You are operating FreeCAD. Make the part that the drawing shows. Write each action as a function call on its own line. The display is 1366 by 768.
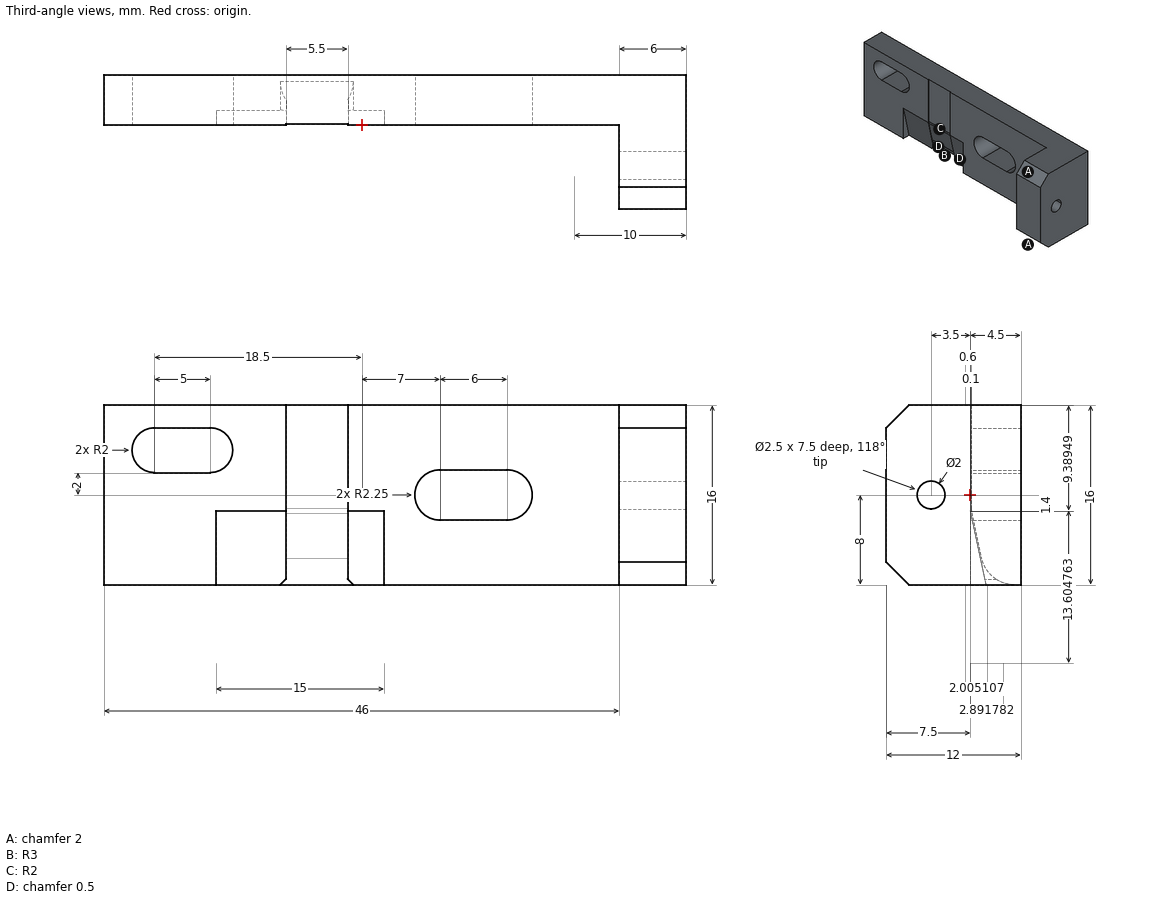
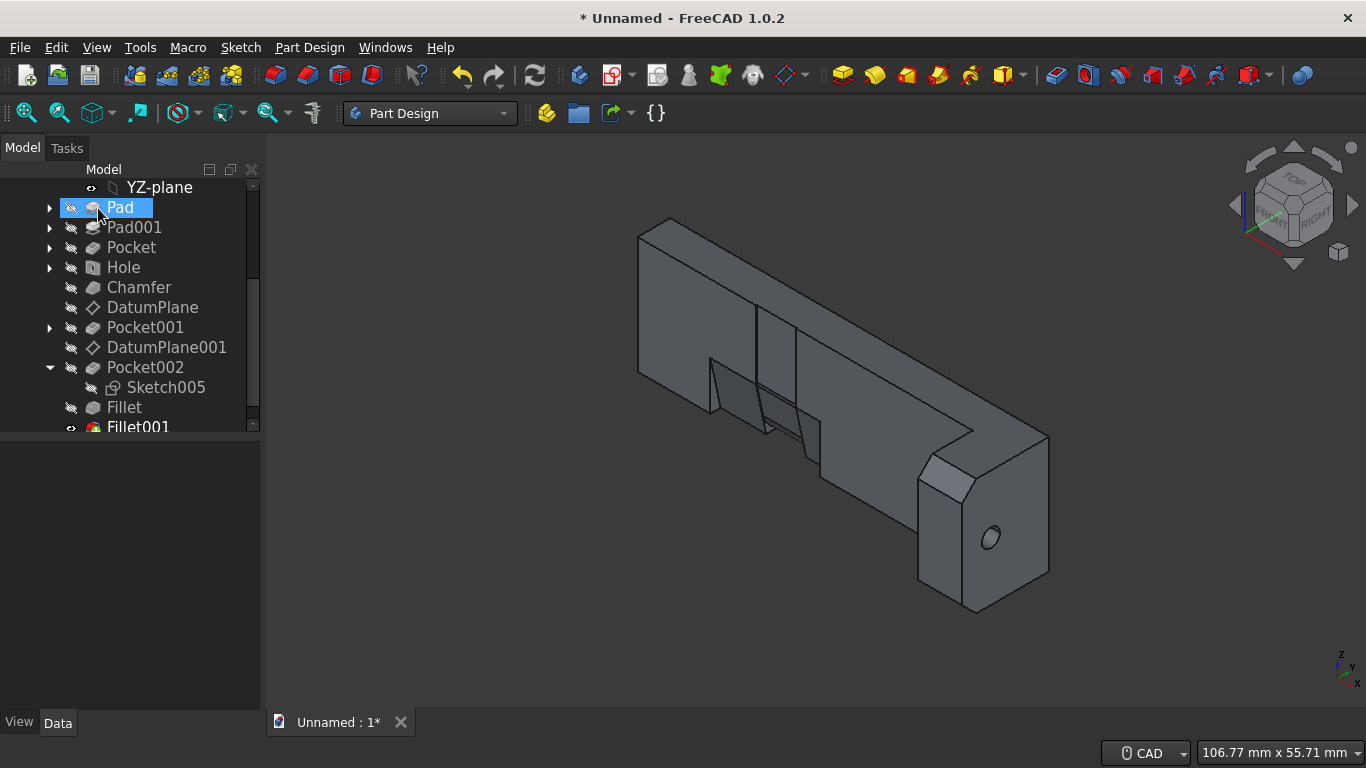
key(4)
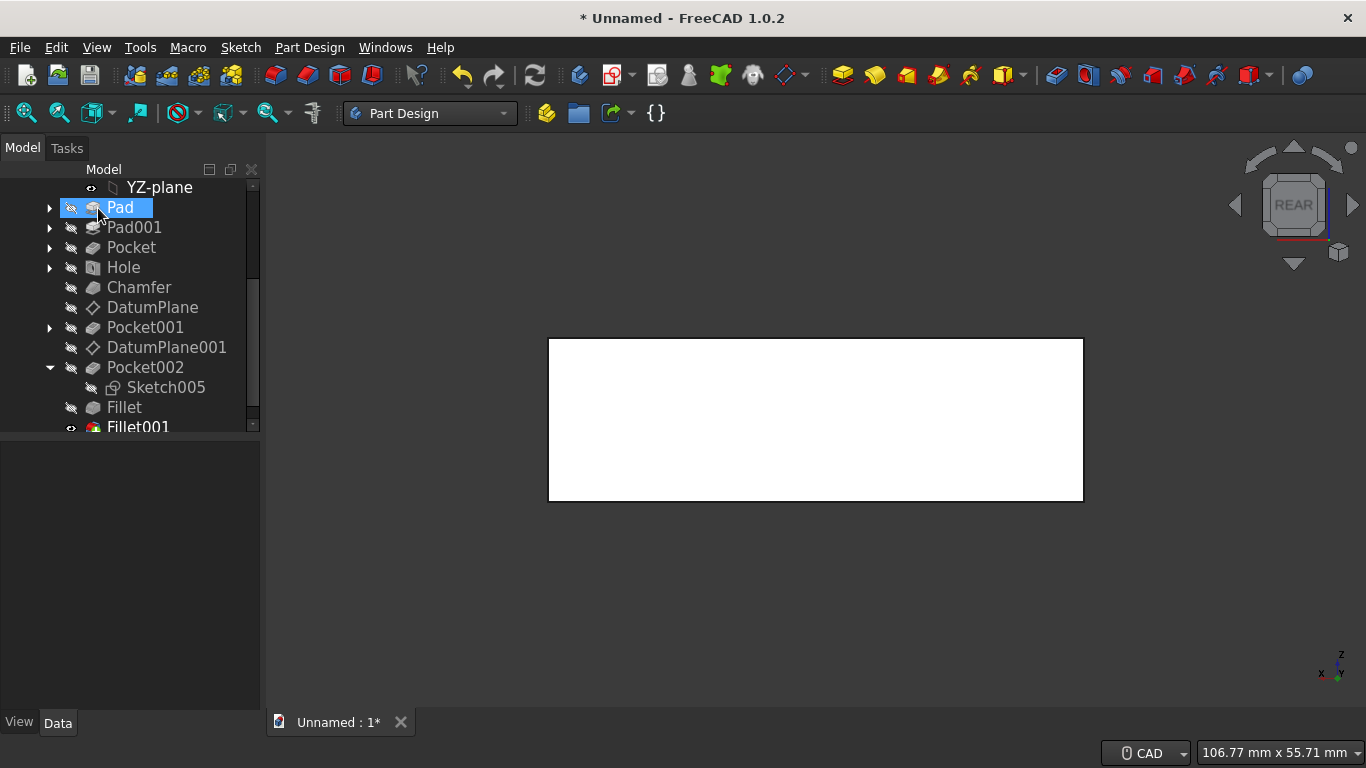
click(663, 419)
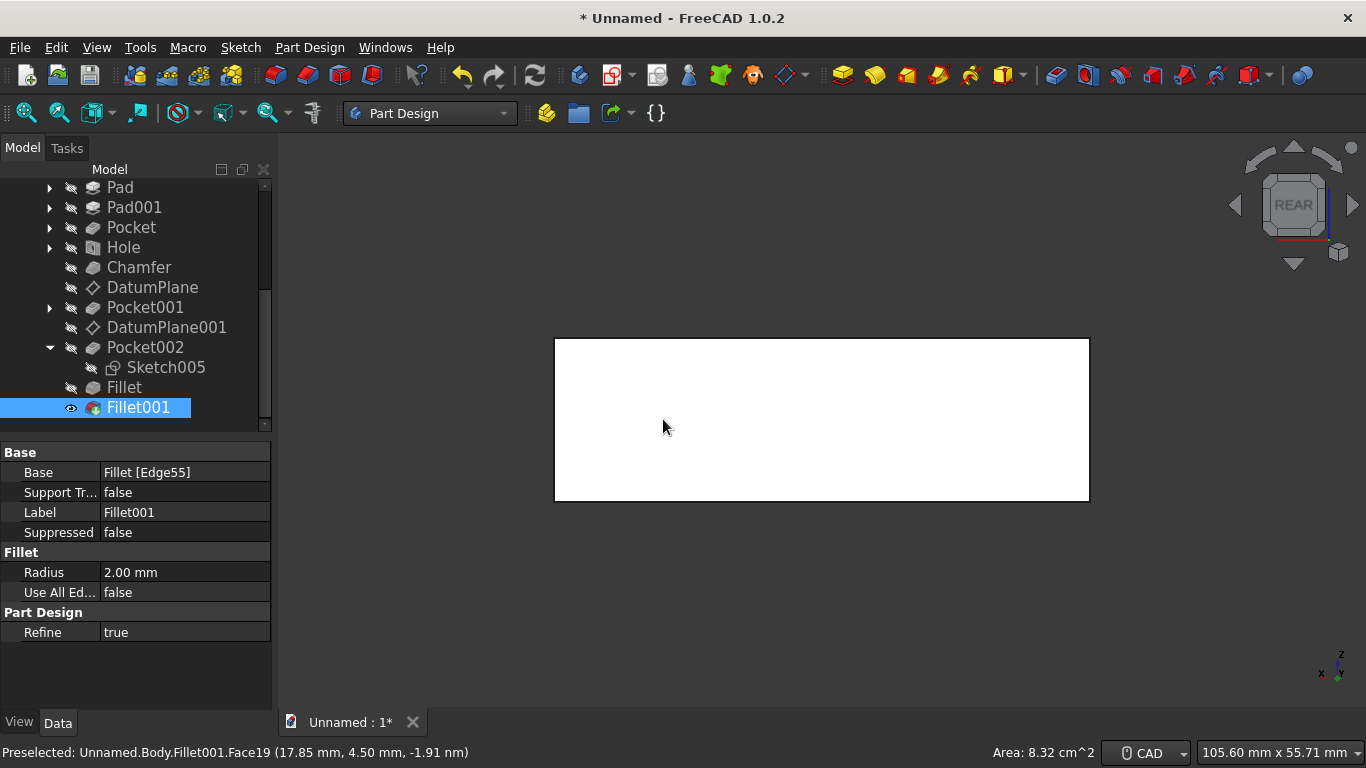
click(612, 76)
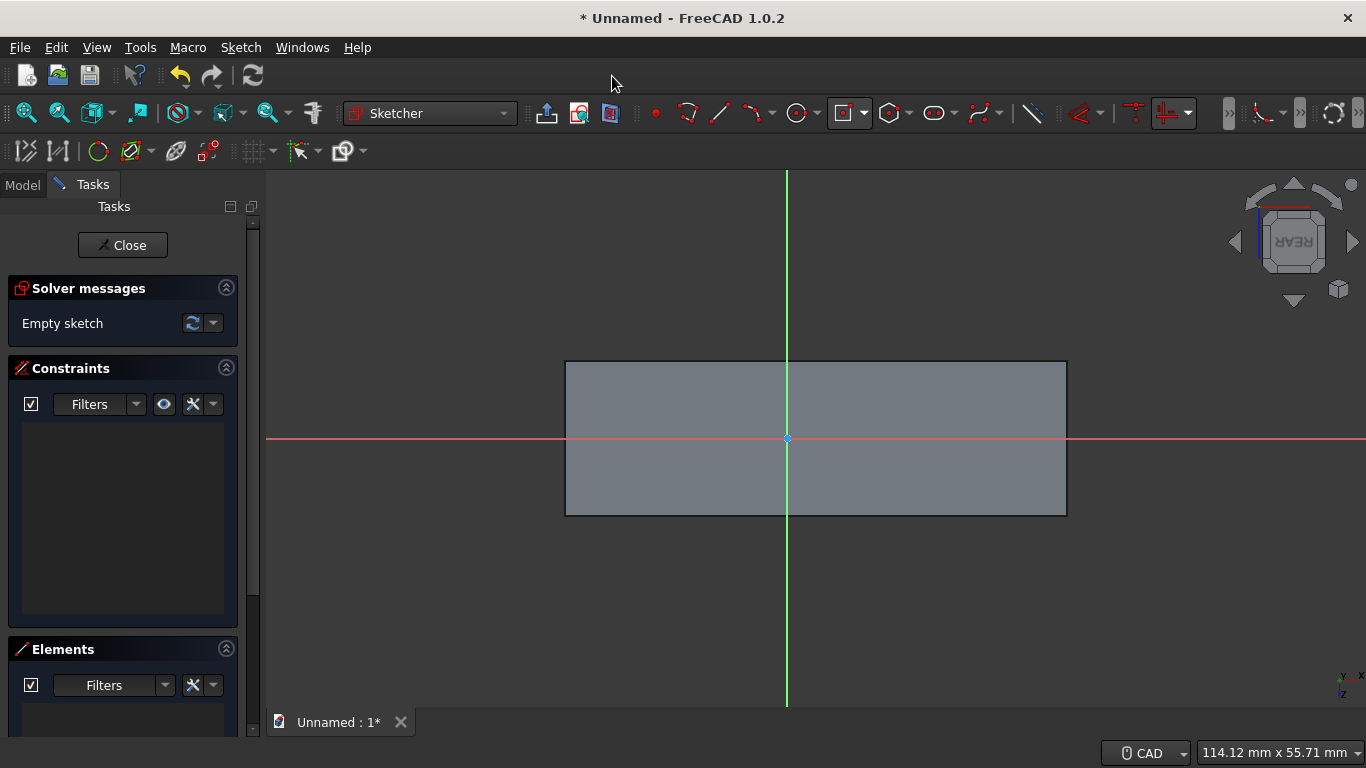
scroll(663, 480, up, 6)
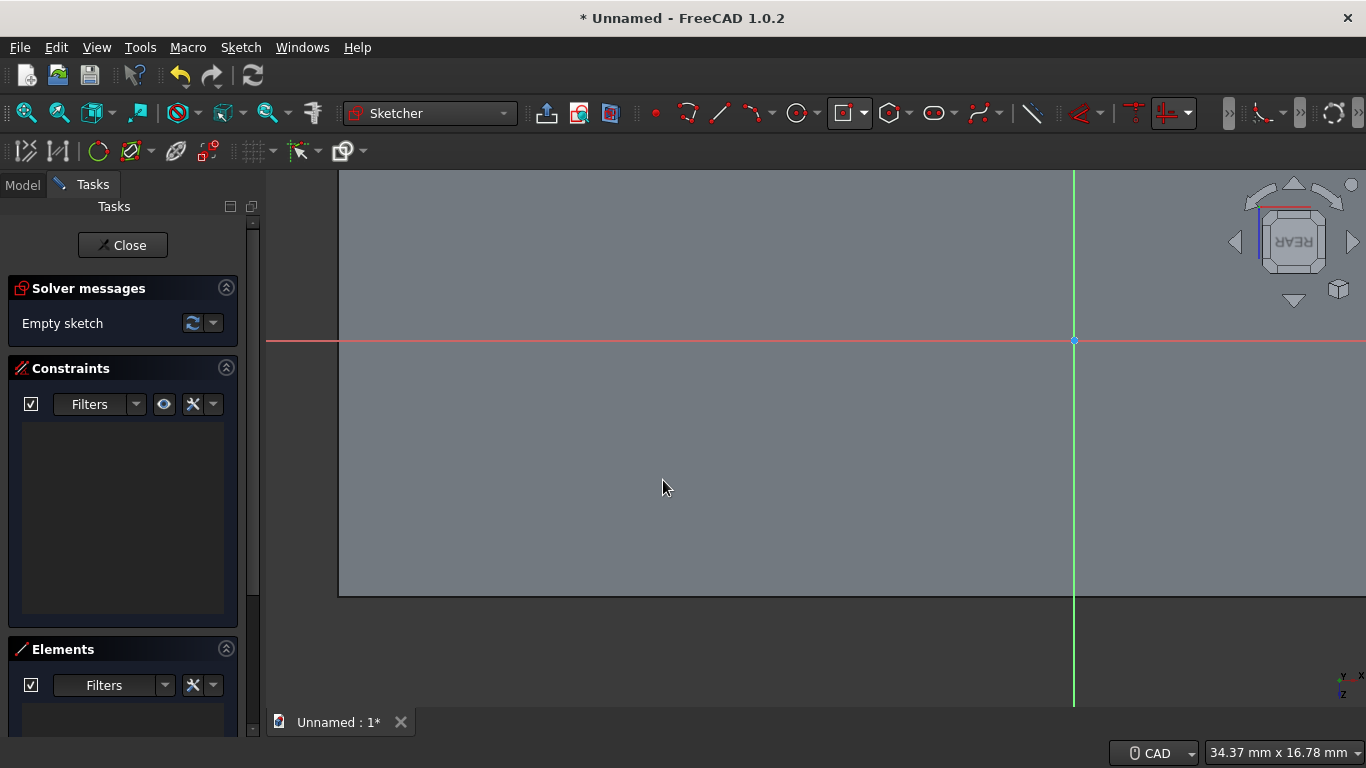
key(g)
key(s)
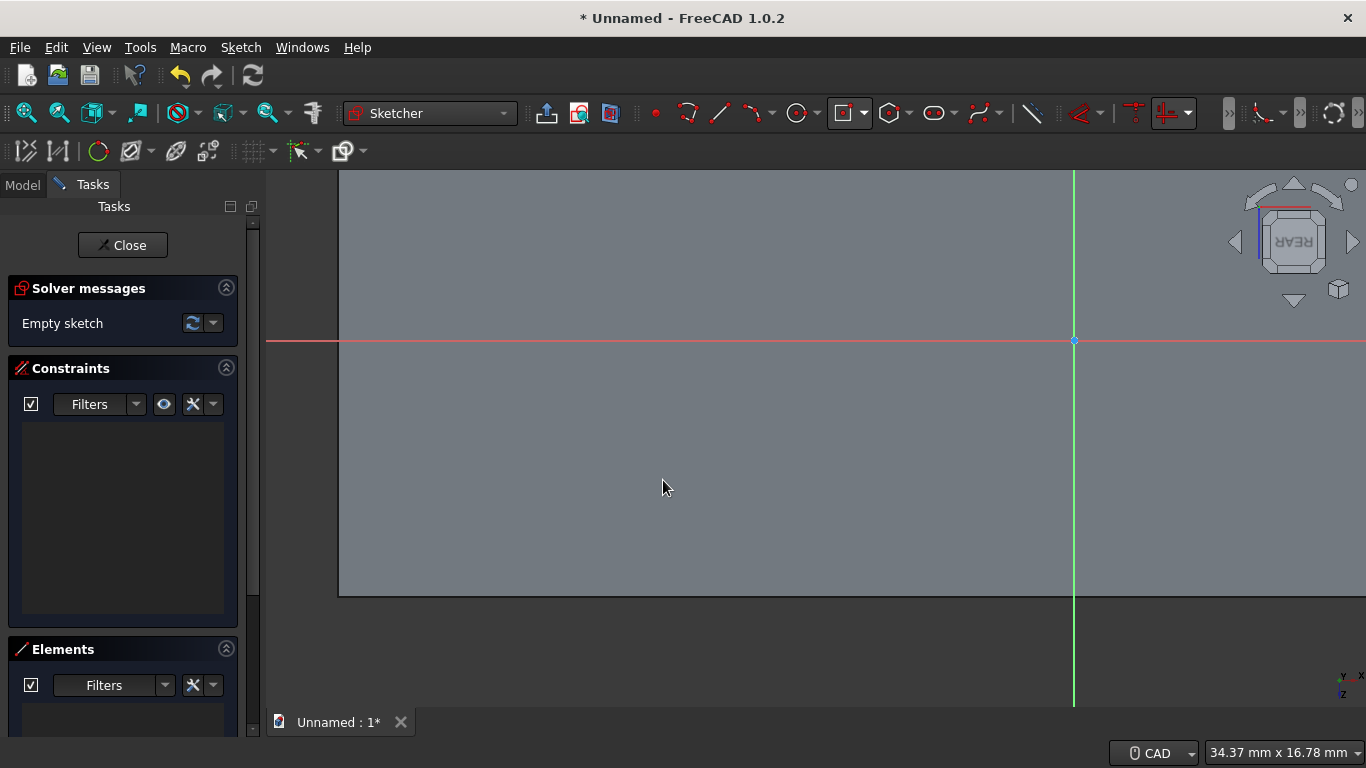
click(482, 469)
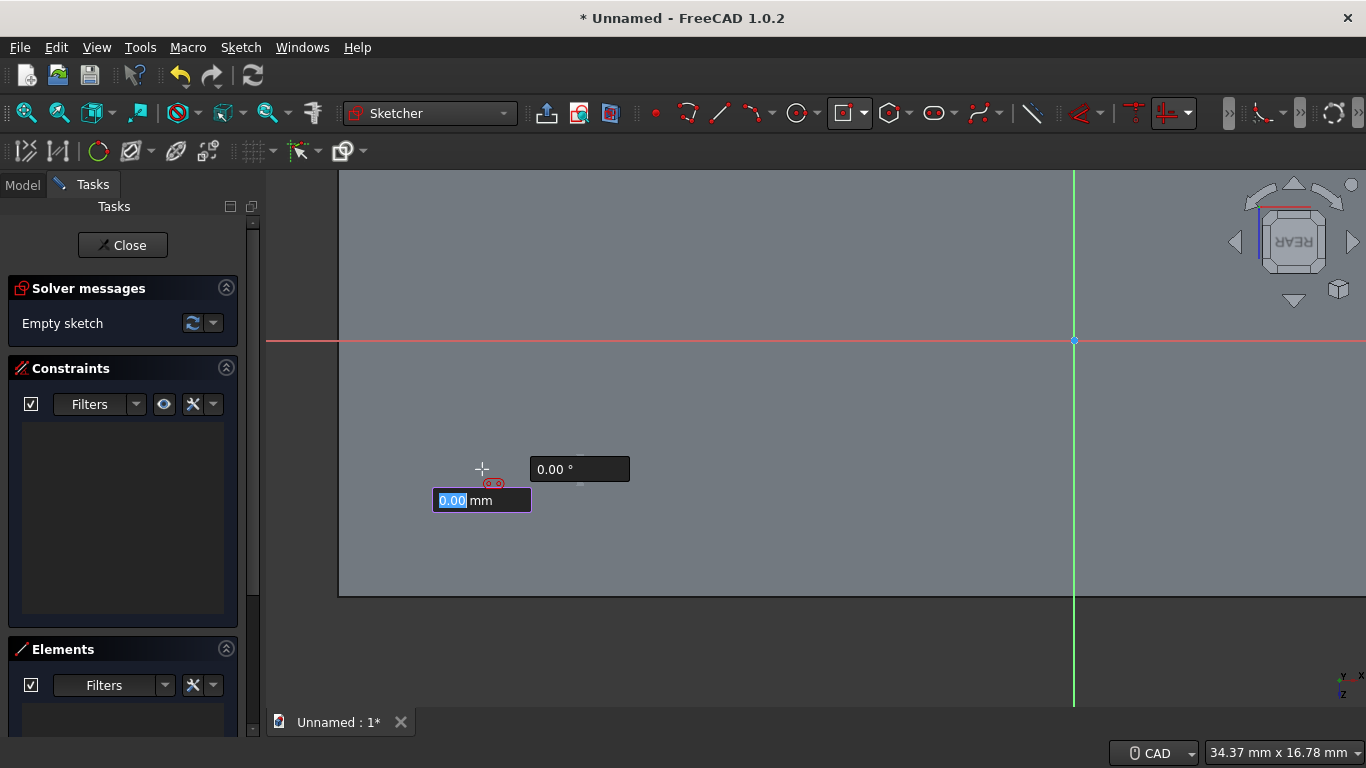
click(642, 469)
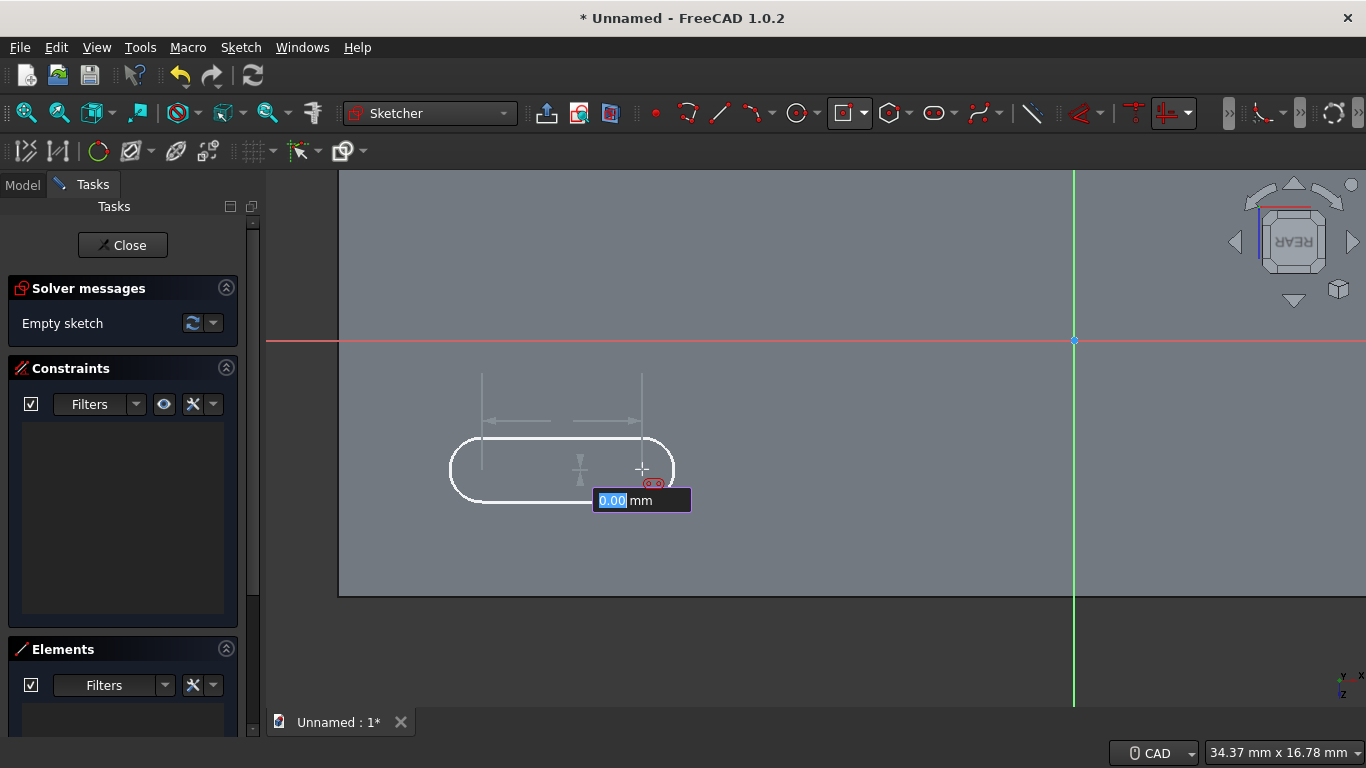
click(562, 405)
key(Escape)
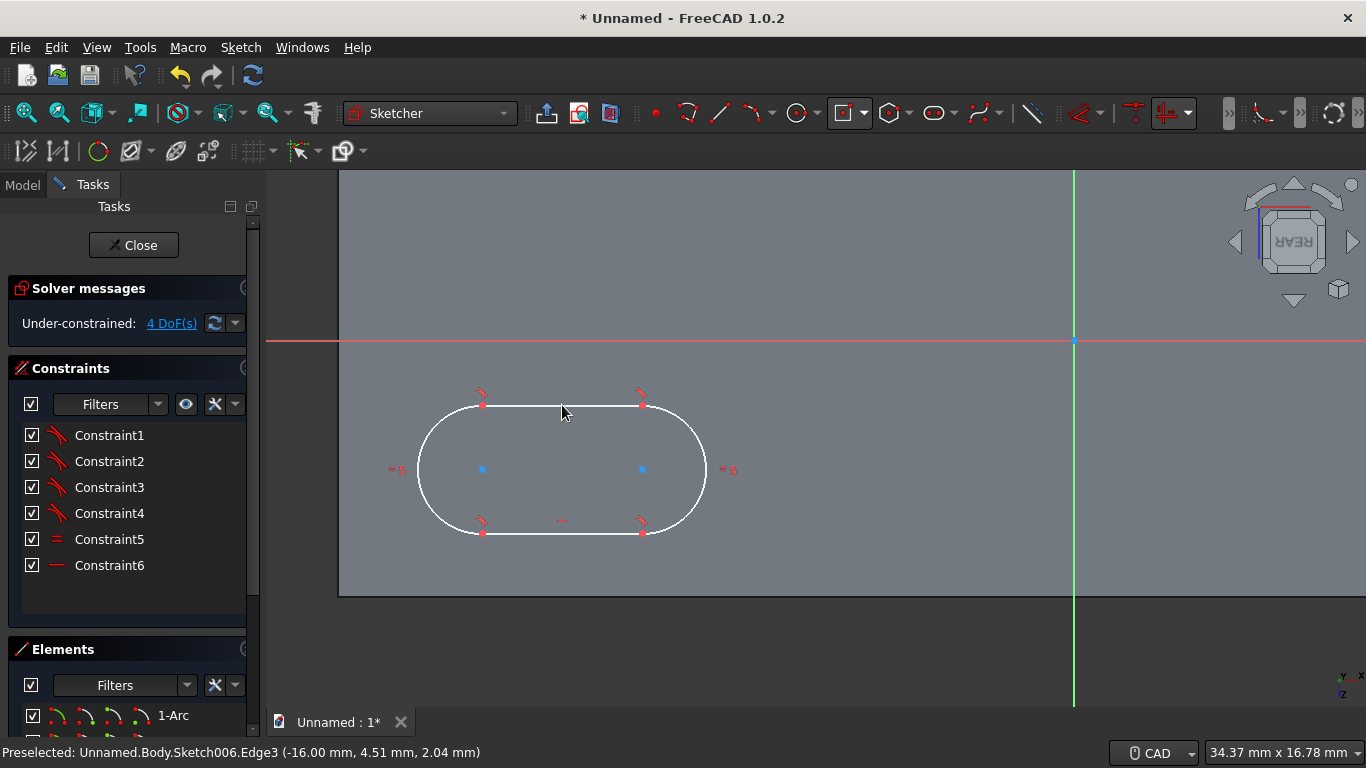
key(d)